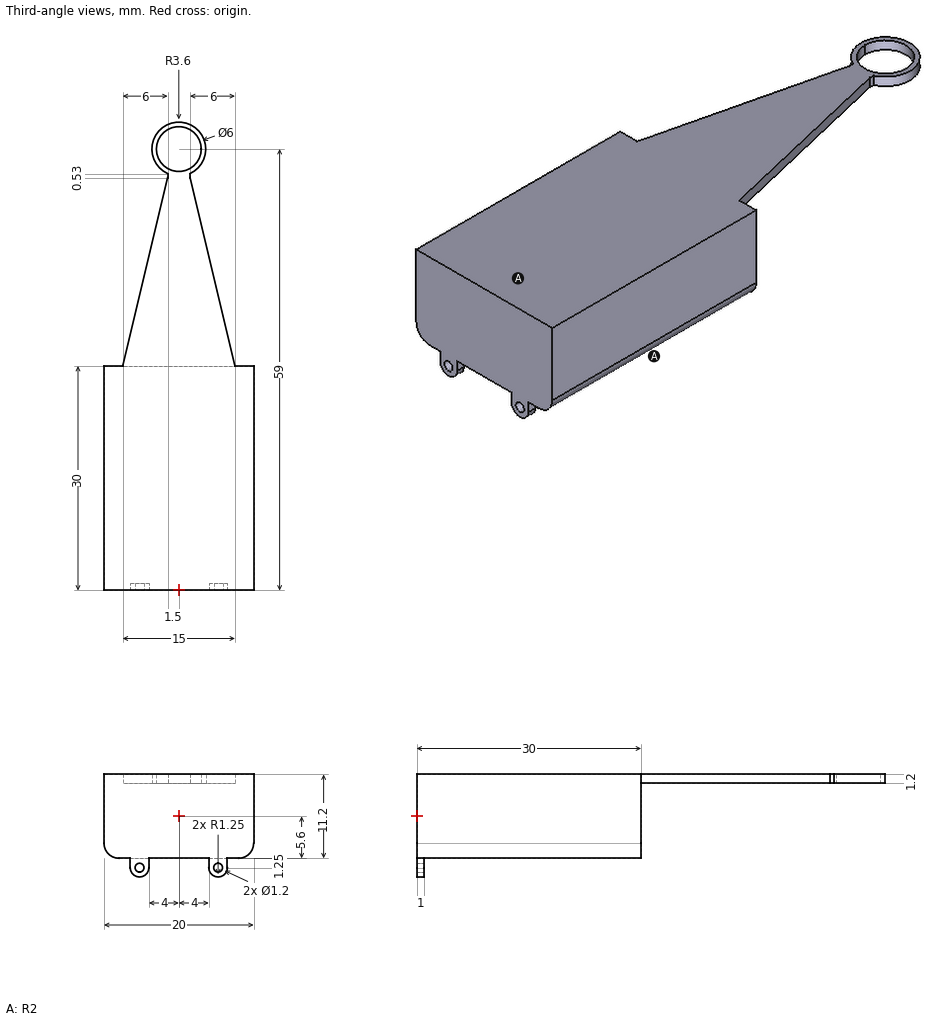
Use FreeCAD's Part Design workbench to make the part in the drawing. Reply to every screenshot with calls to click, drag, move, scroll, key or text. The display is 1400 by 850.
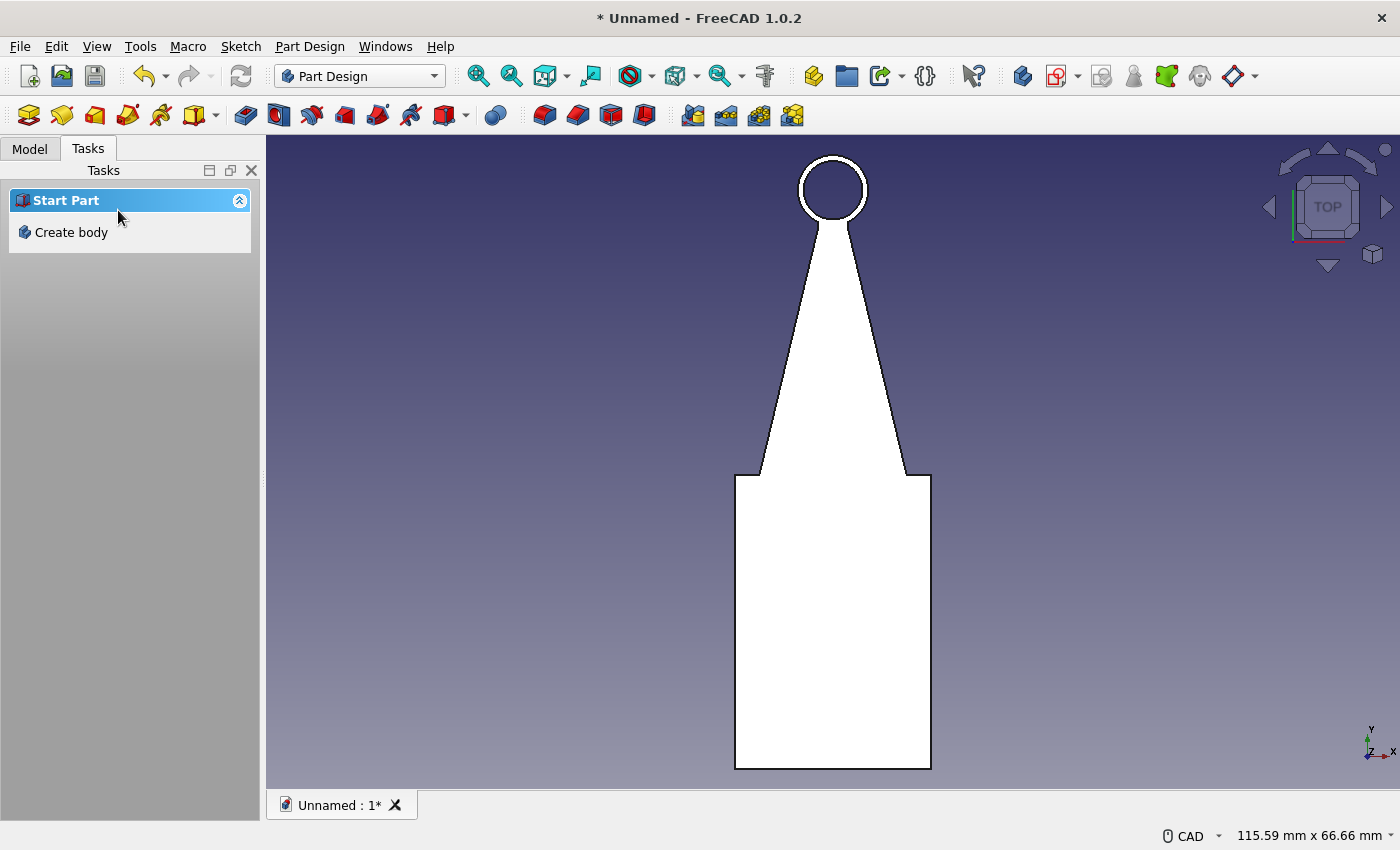
key(1)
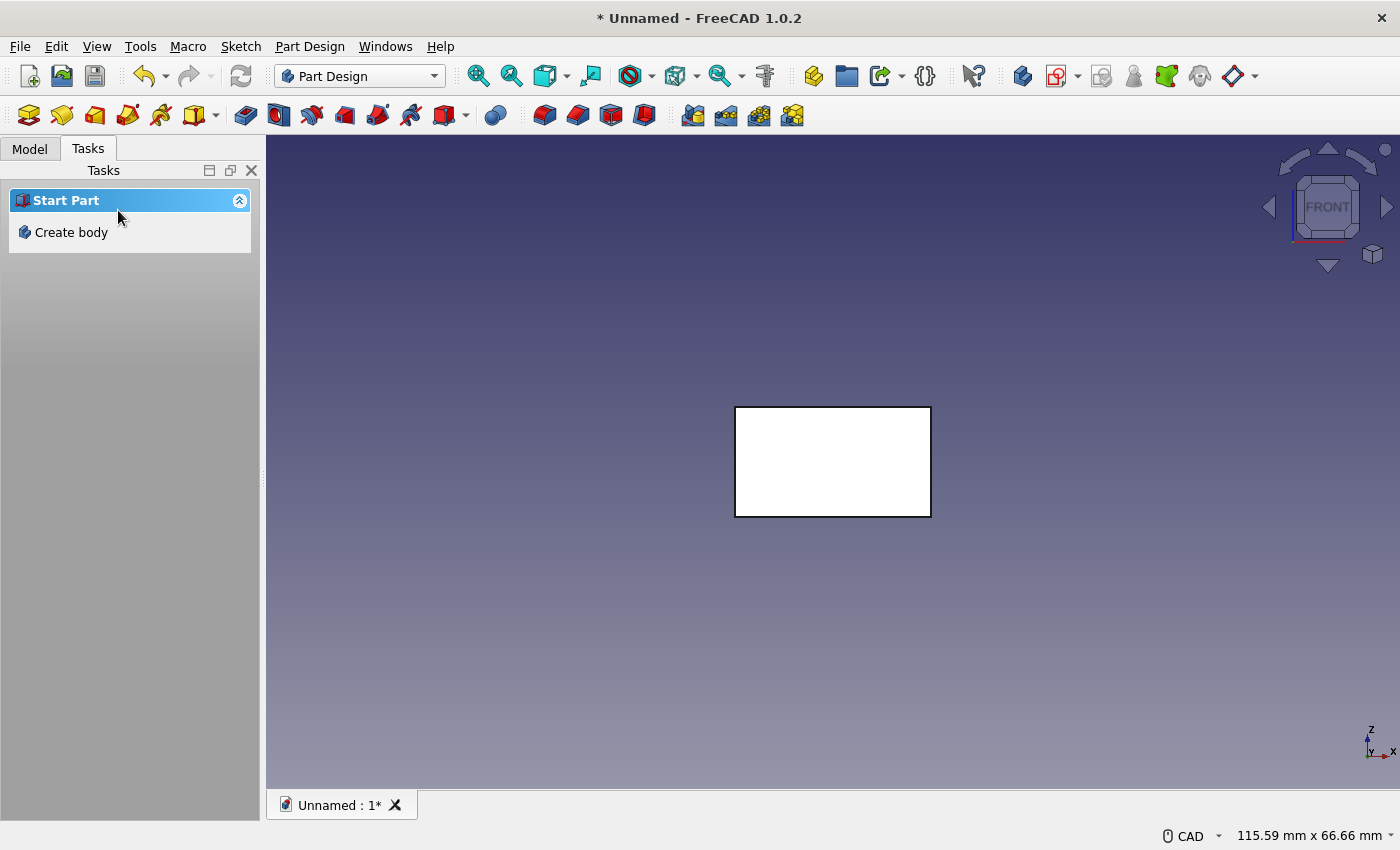
key(v)
key(f)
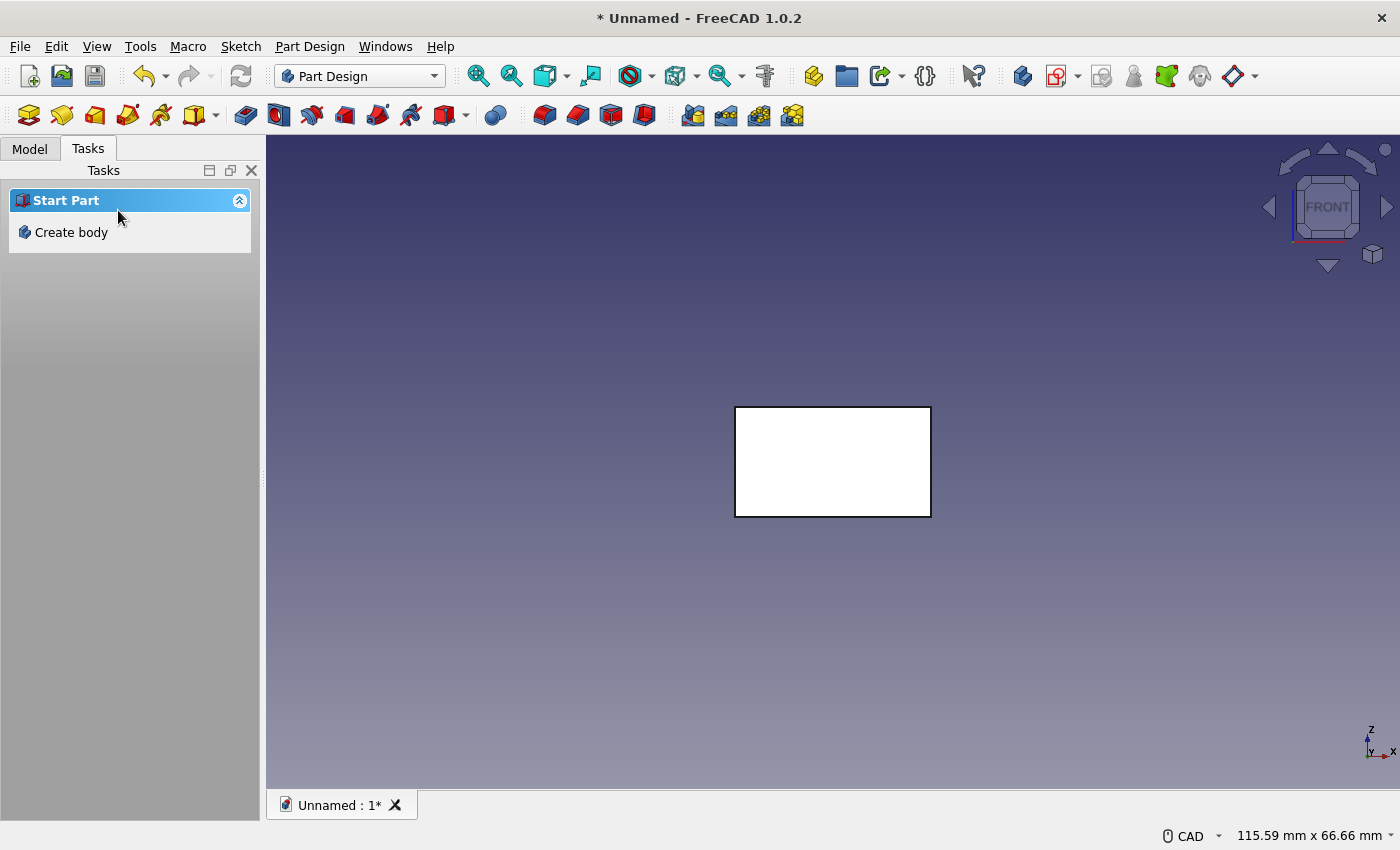
key(3)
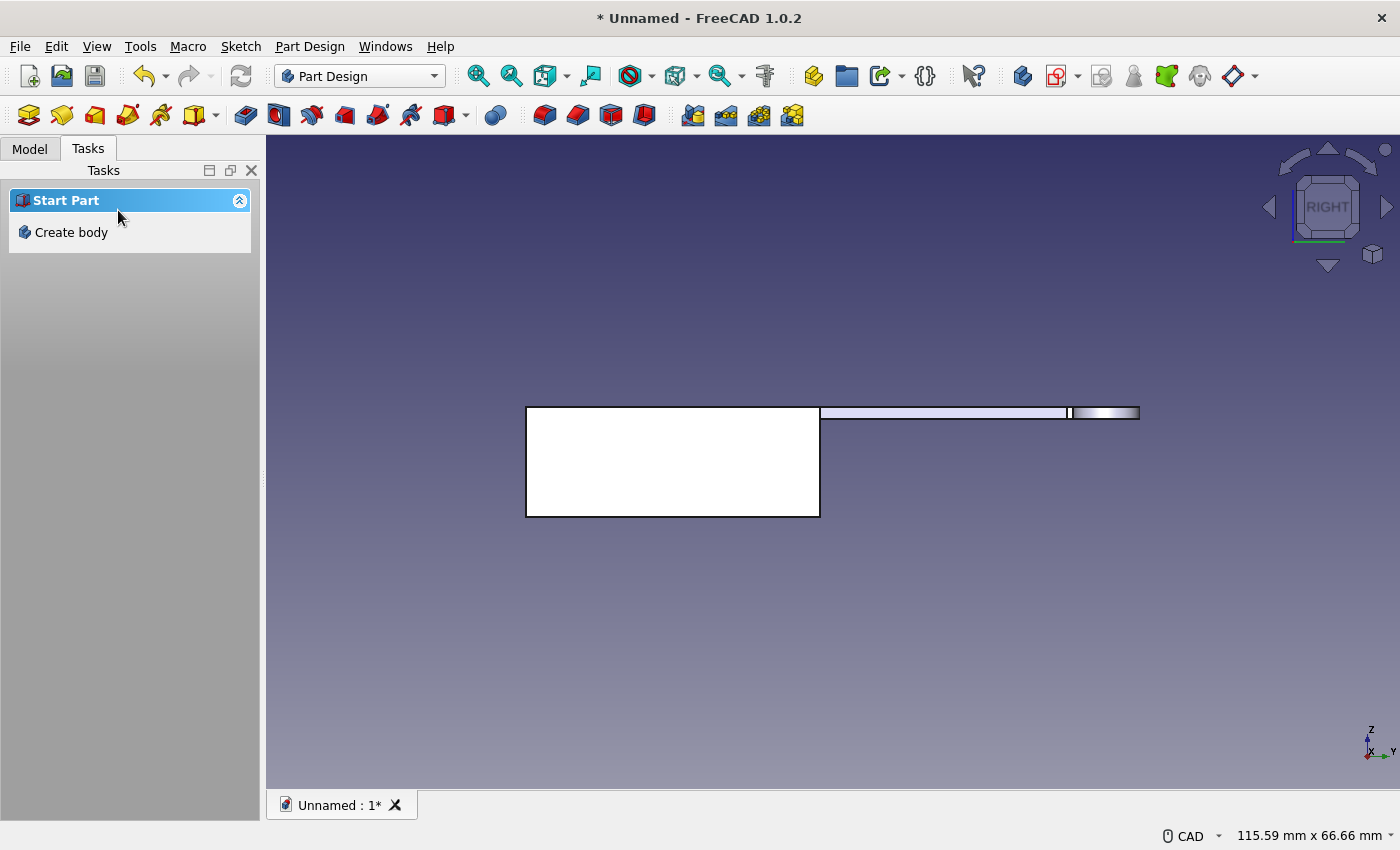
click(673, 516)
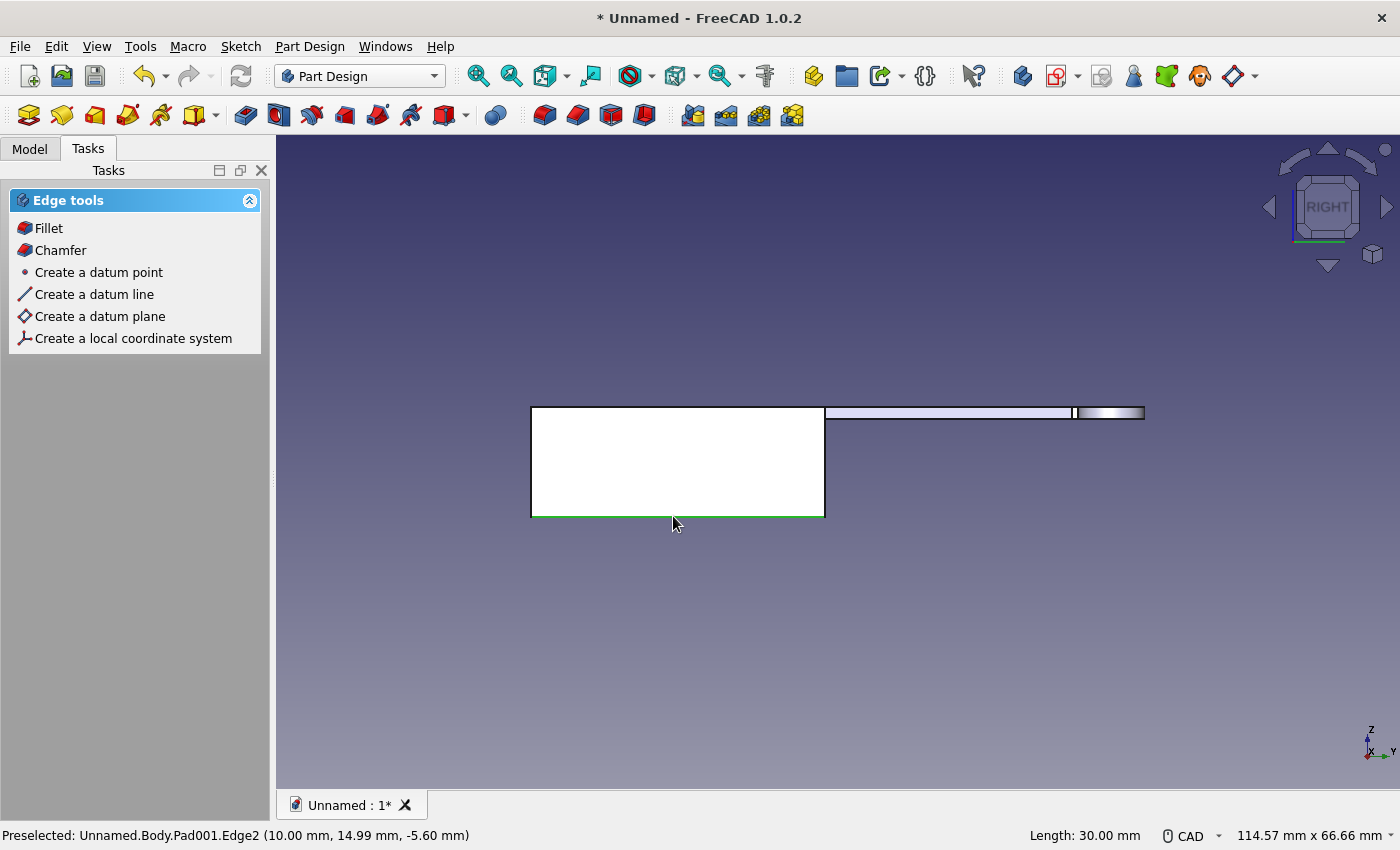
key(5)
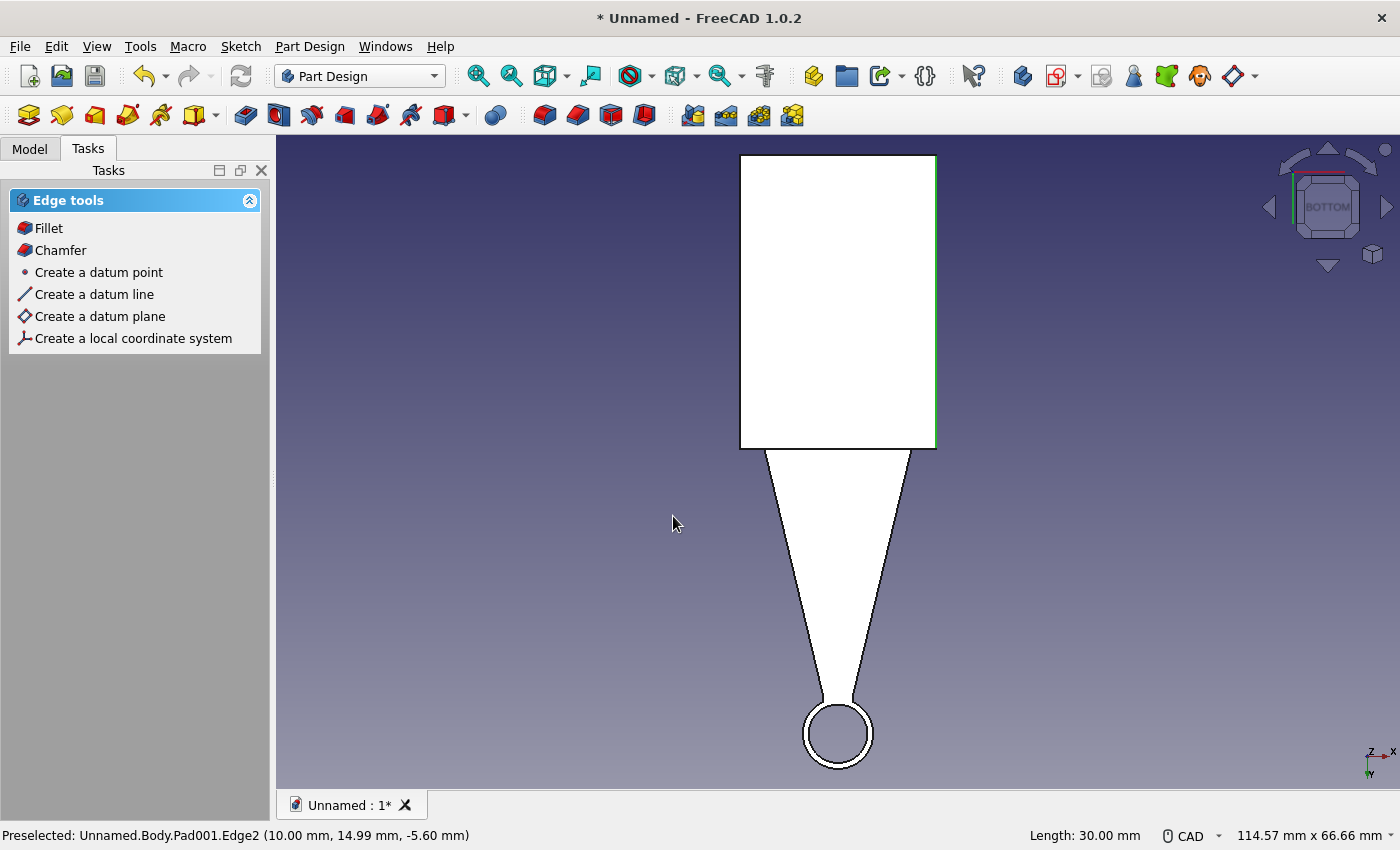
click(740, 301, ctrl)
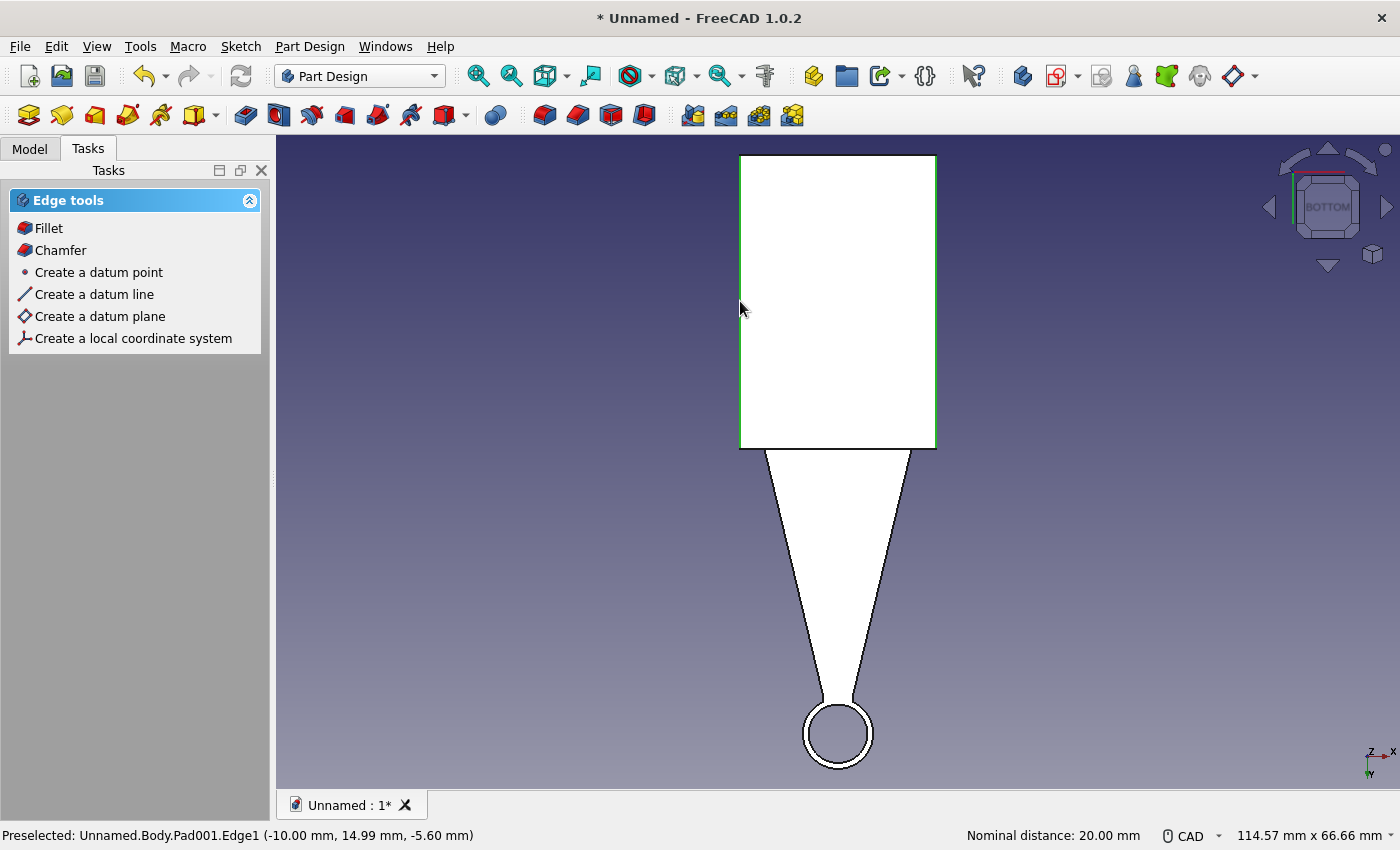
click(545, 116)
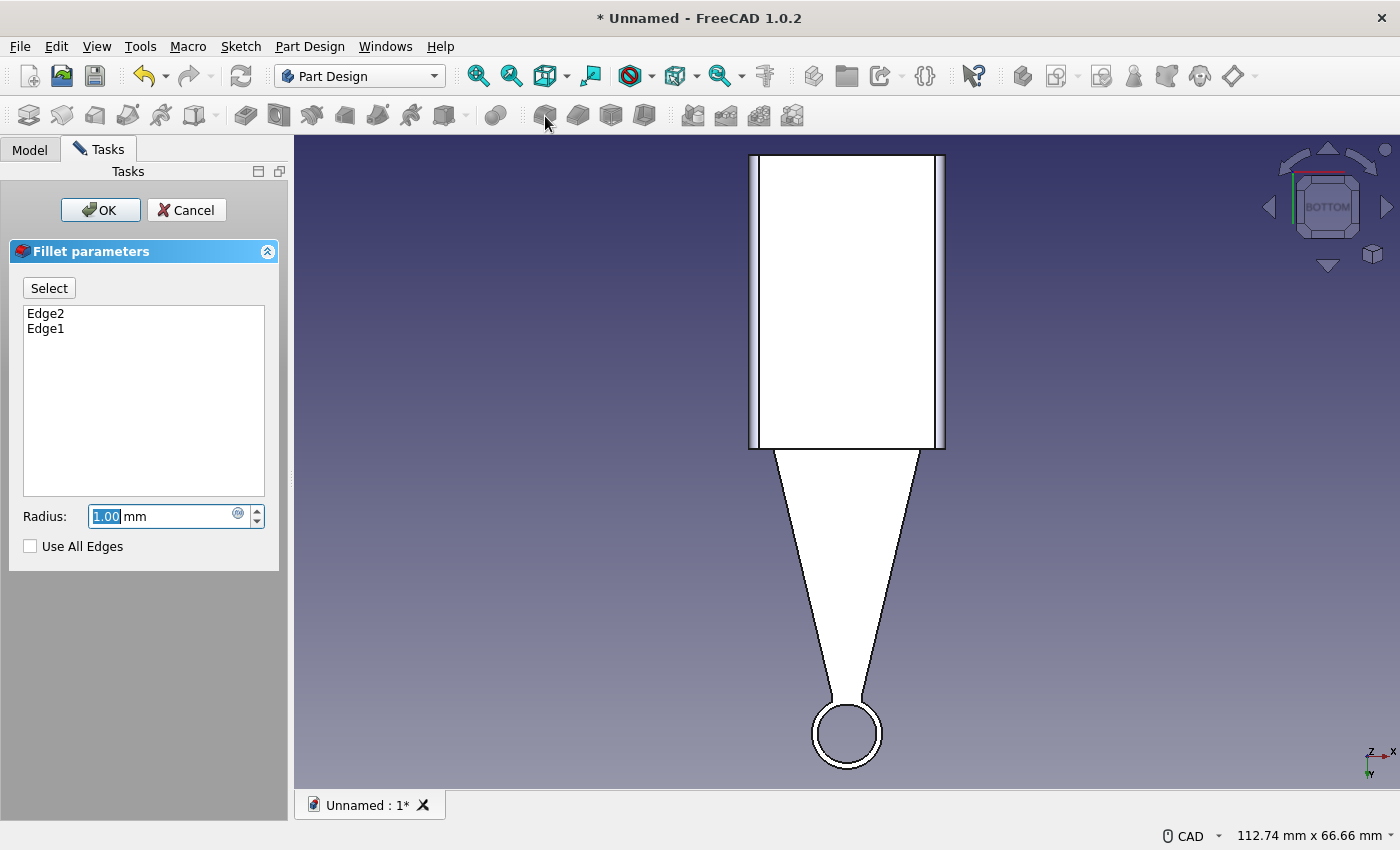
text(2)
key(Tab)